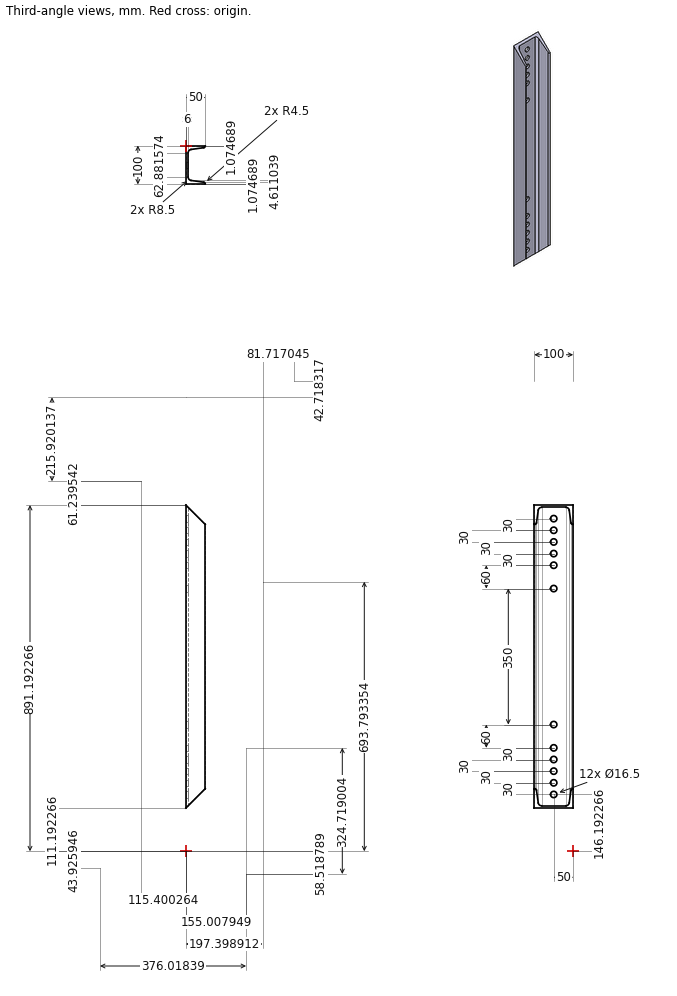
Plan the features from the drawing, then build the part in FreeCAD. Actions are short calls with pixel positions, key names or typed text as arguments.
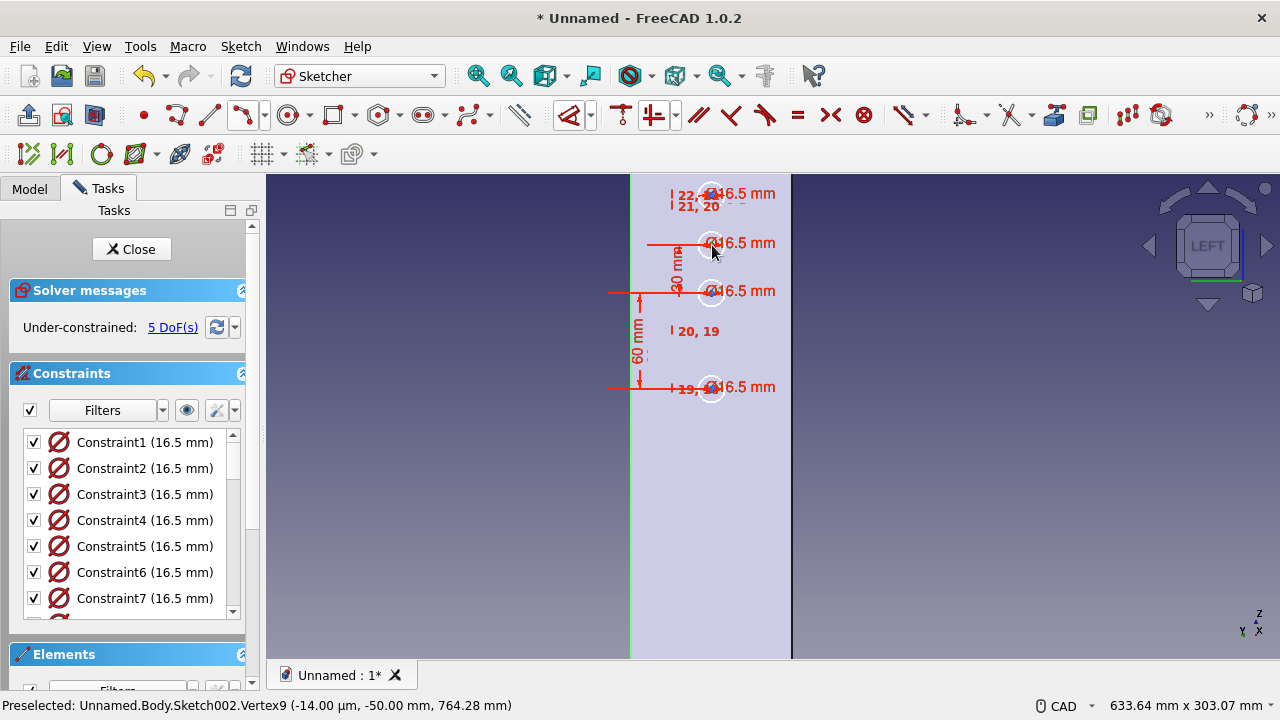
scroll(711, 325, down, 8)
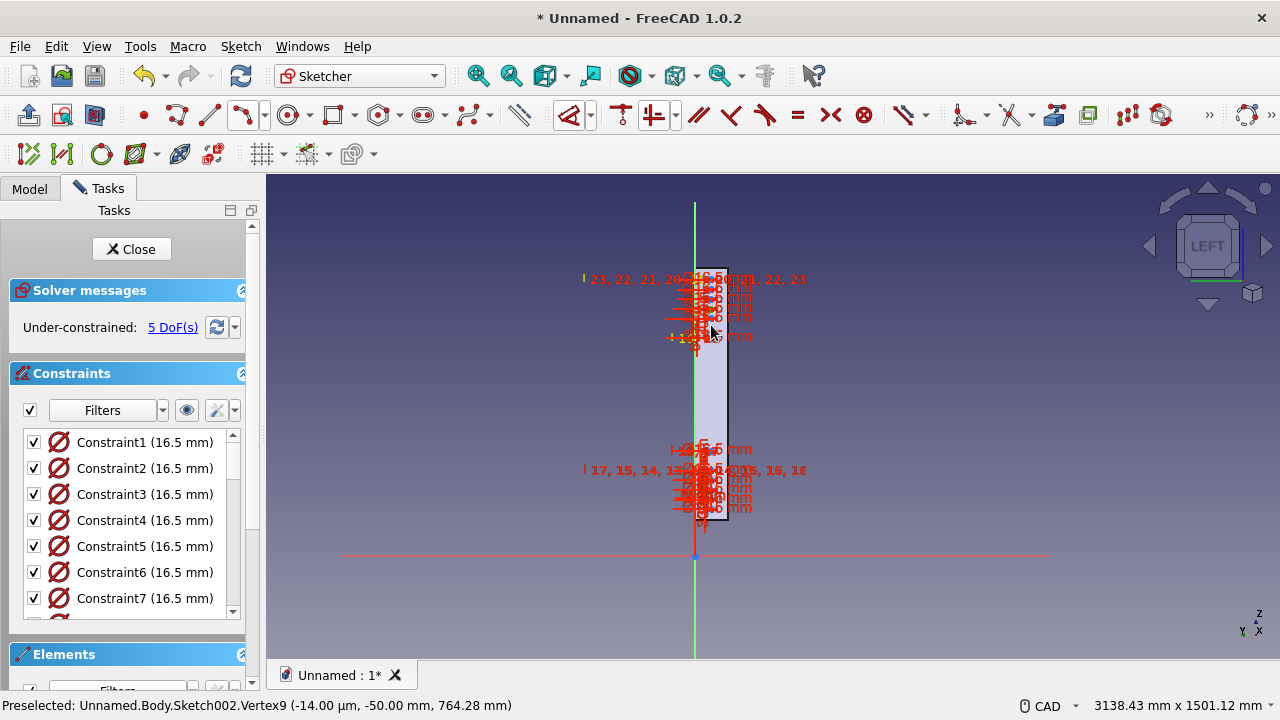
scroll(711, 299, up, 8)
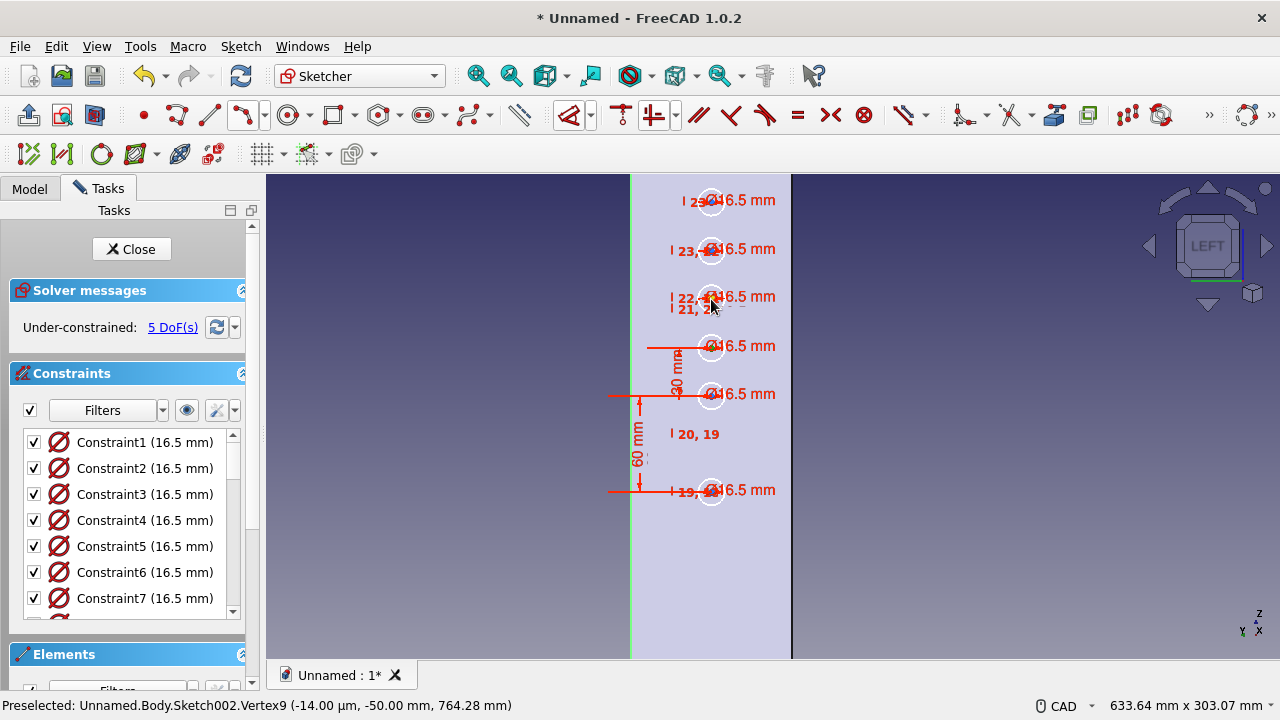
click(712, 299)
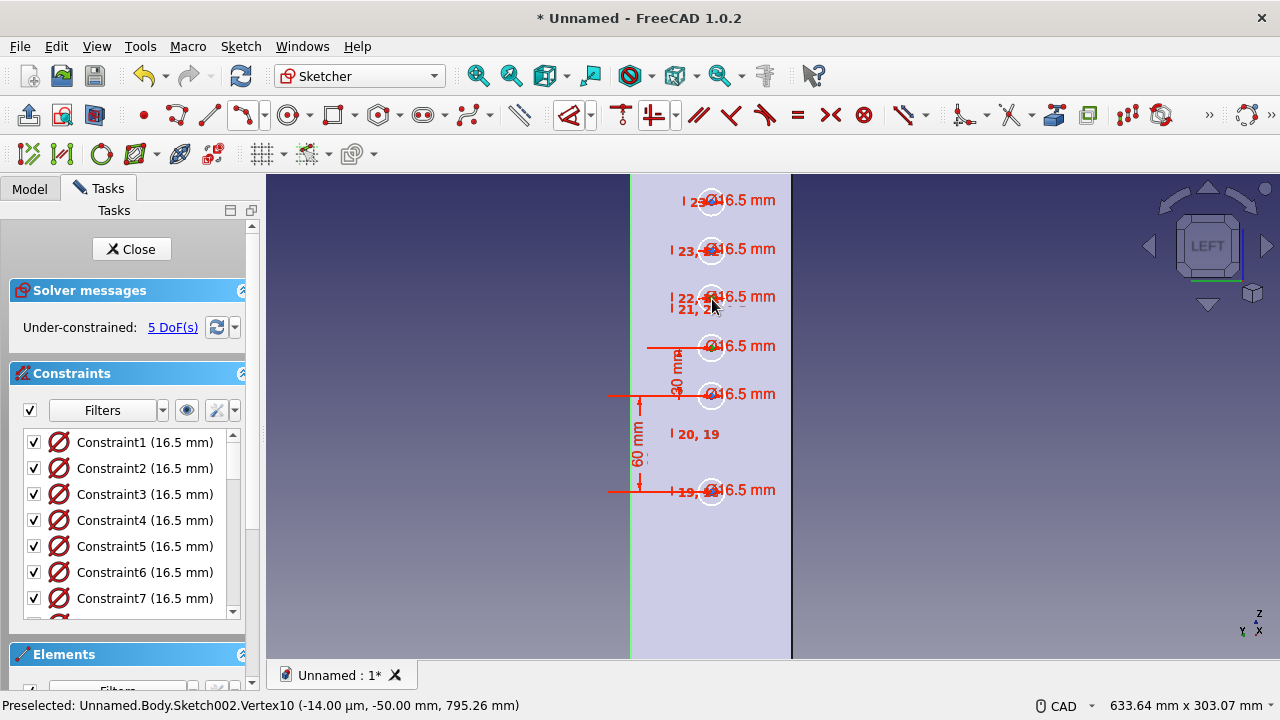
click(590, 116)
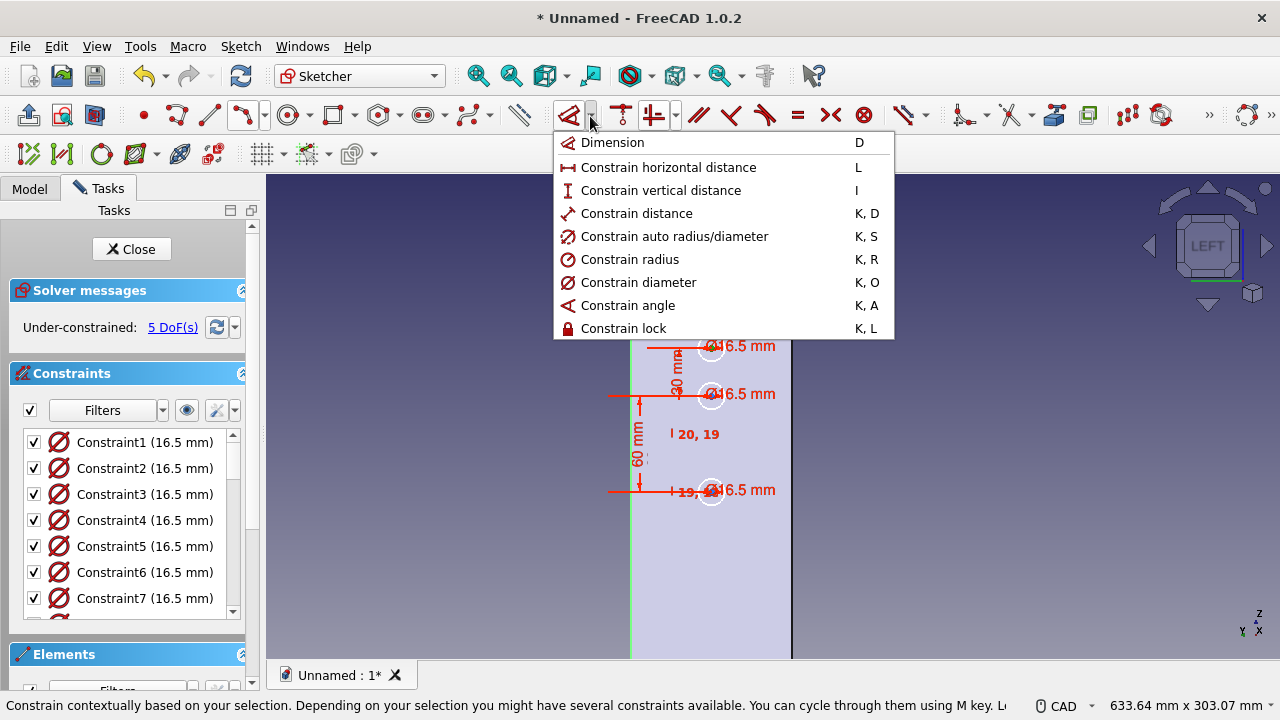
click(724, 190)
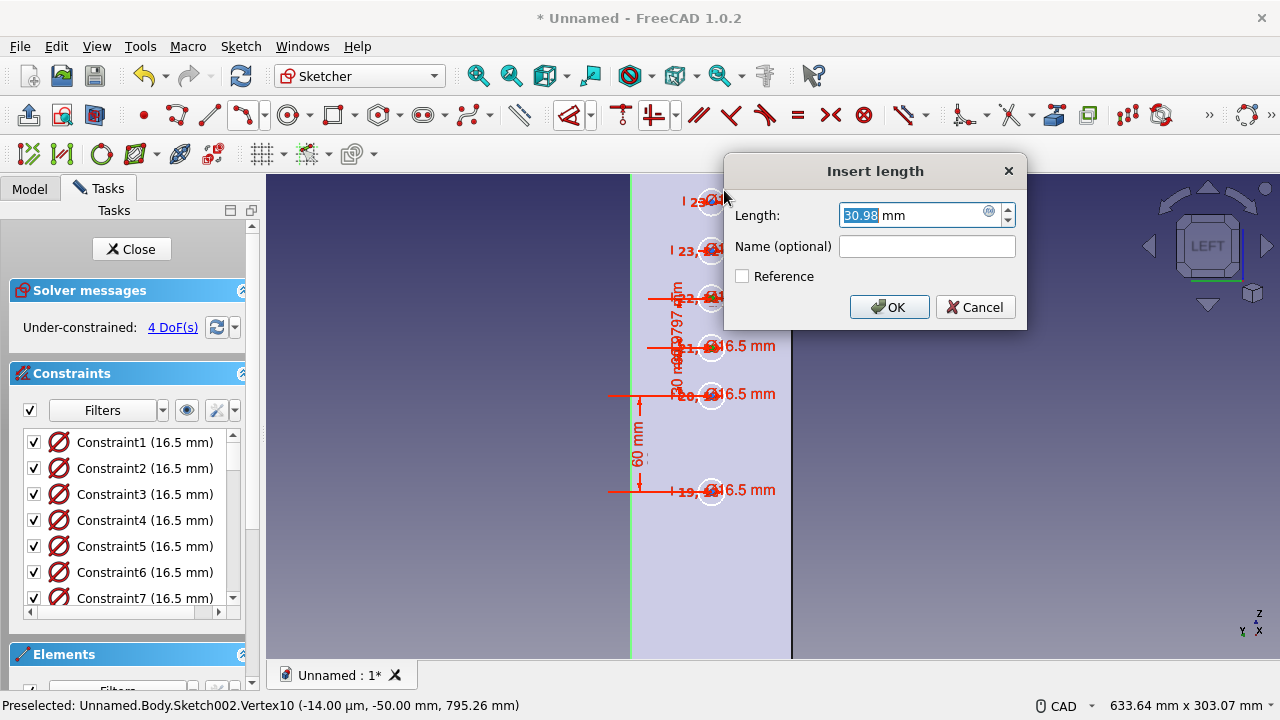
text(30)
key(Return)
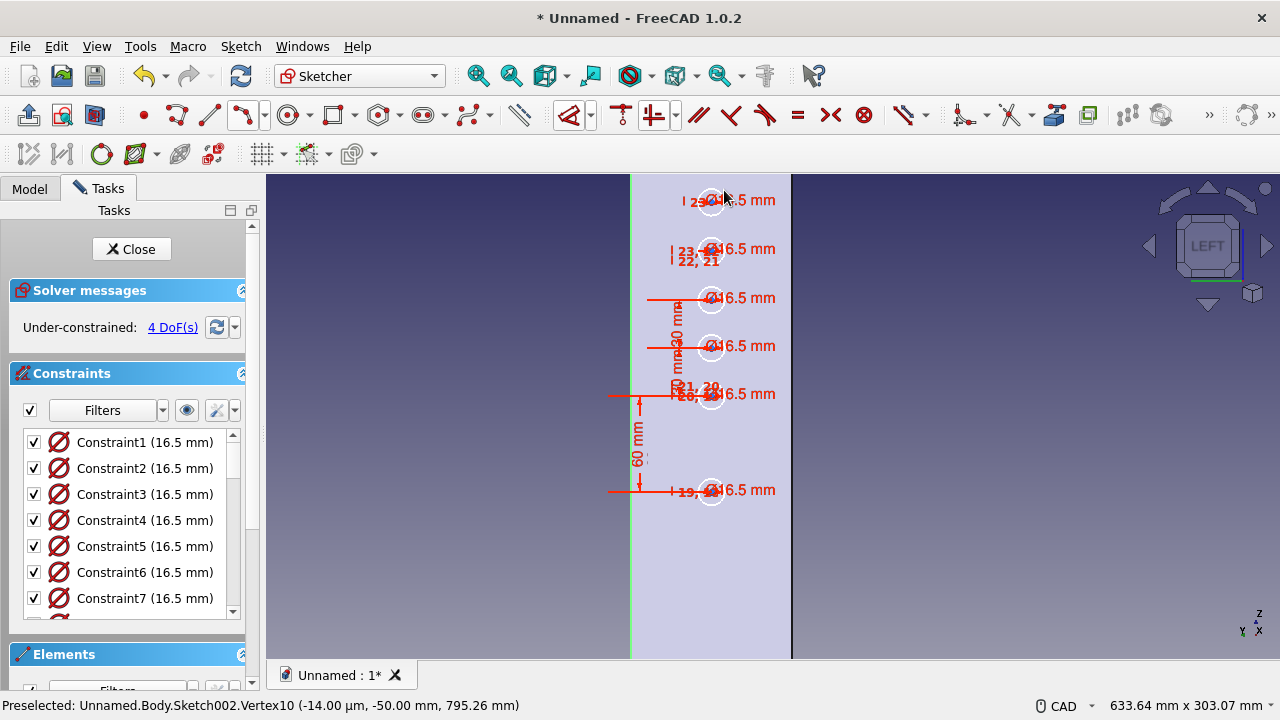
click(712, 300)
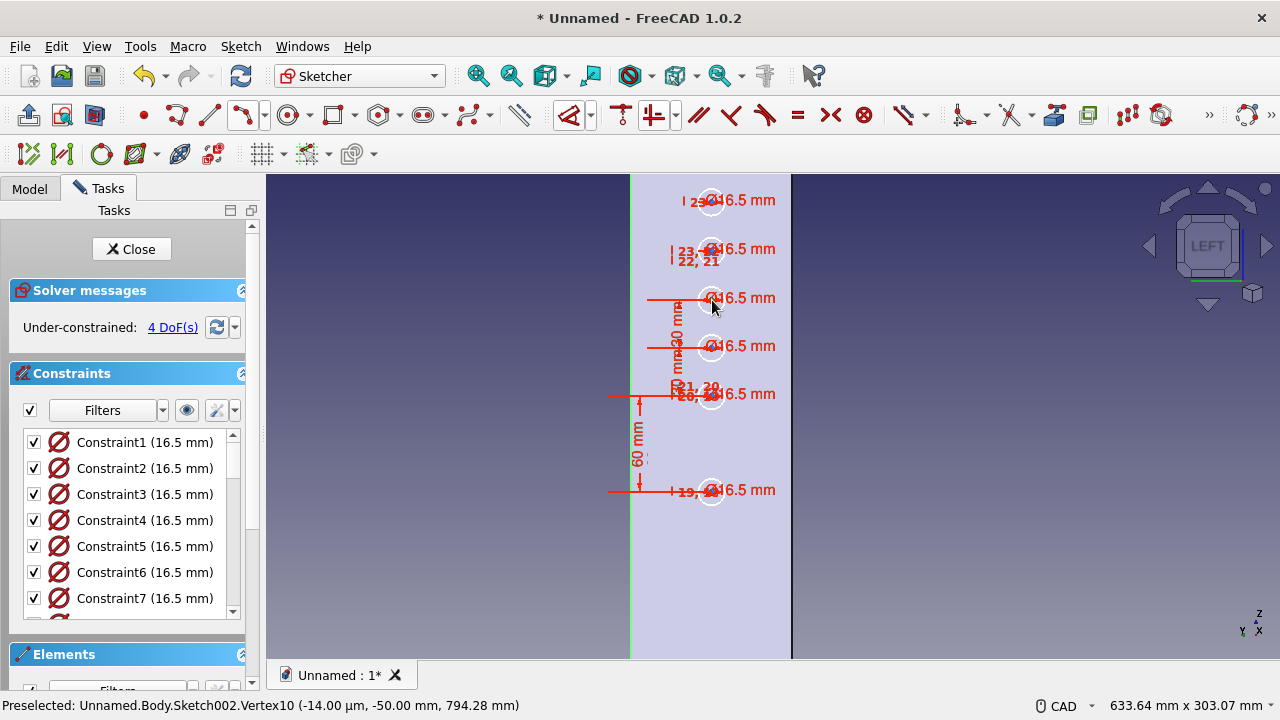
click(712, 251)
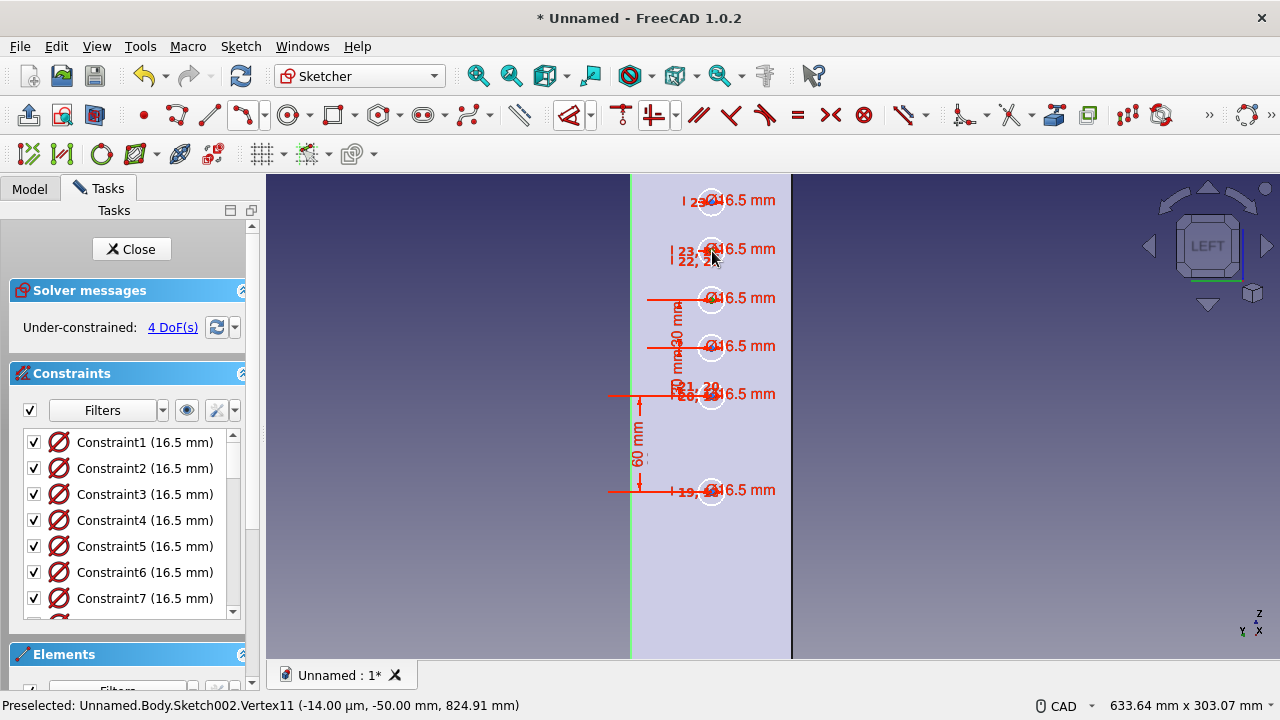
click(590, 116)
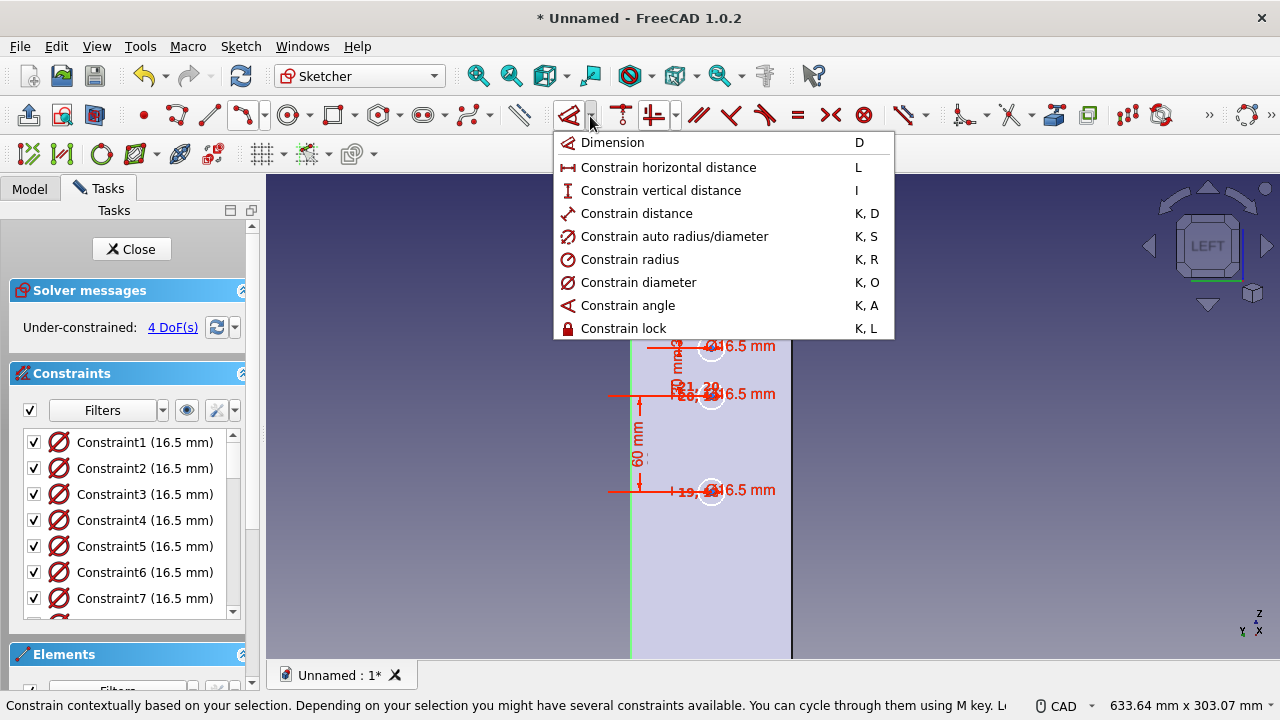
click(724, 190)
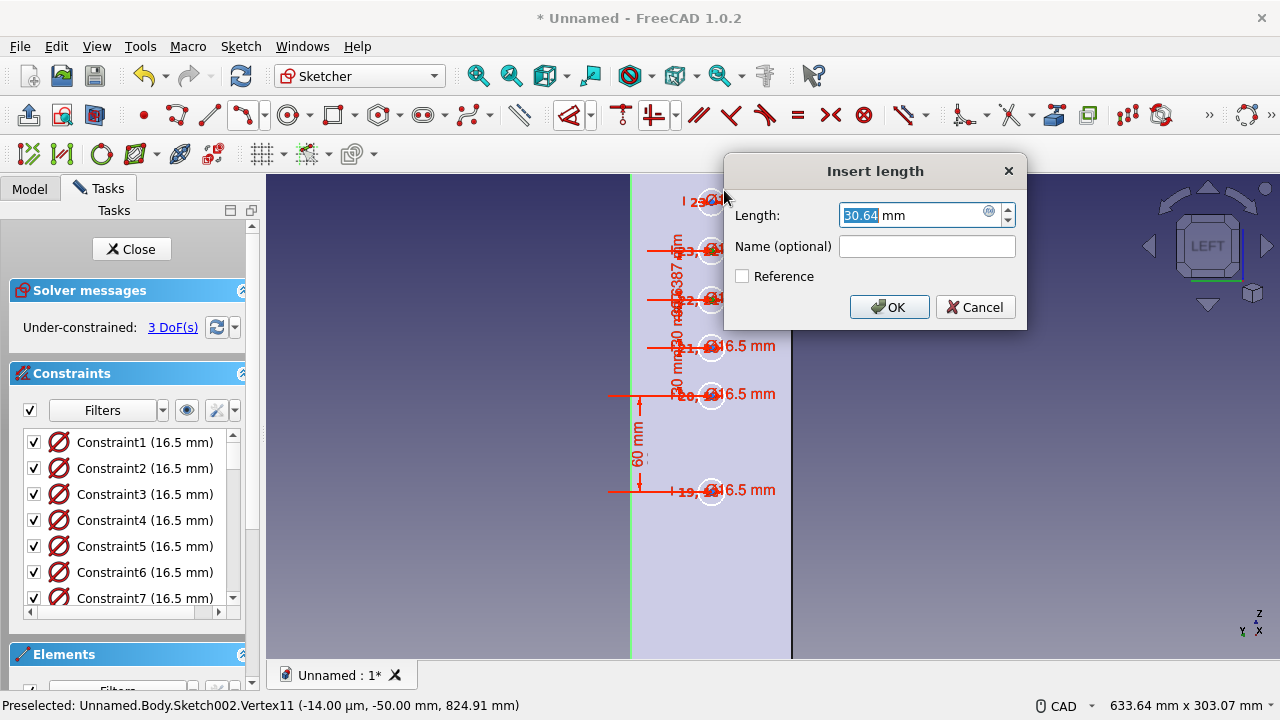
text(30)
key(Return)